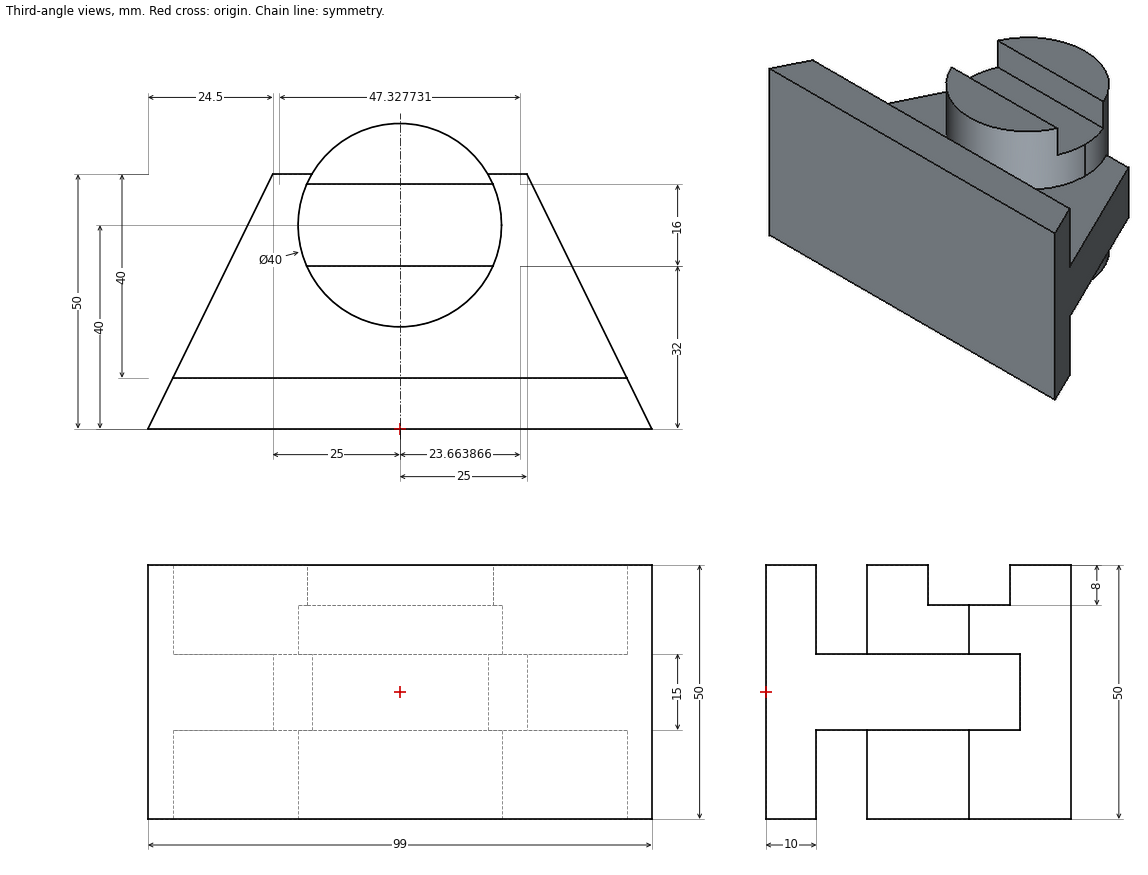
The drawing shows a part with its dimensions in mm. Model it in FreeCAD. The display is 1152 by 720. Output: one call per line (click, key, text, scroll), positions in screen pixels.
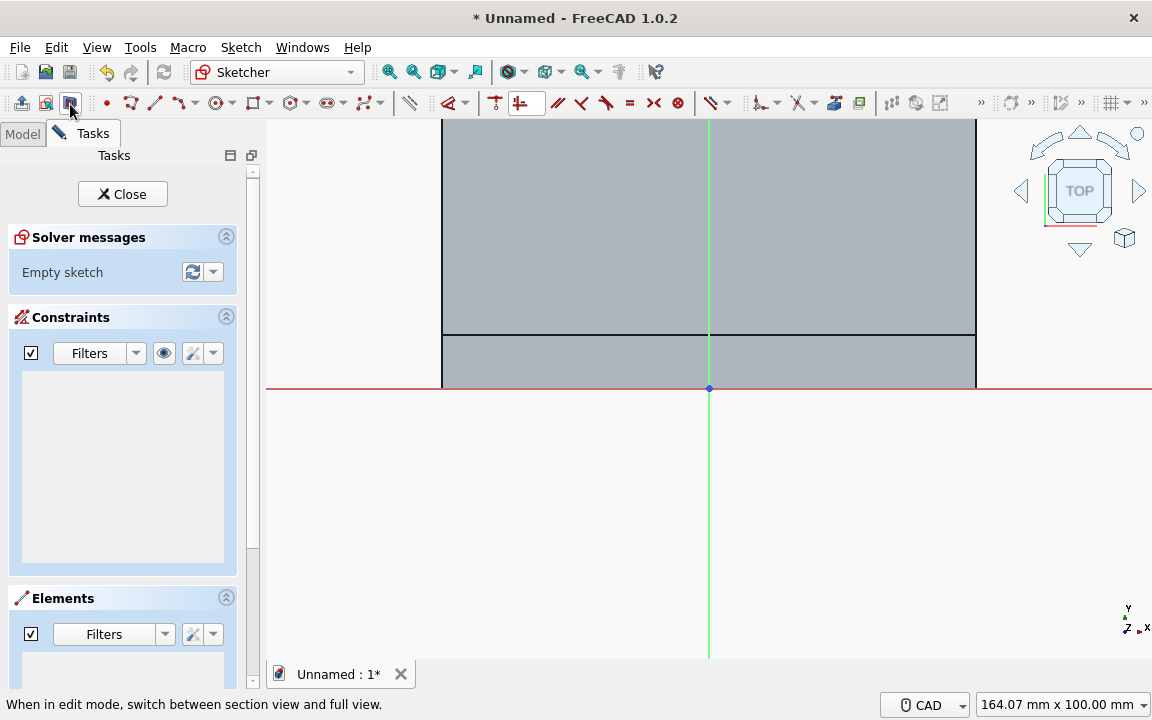
scroll(331, 631, down, 1)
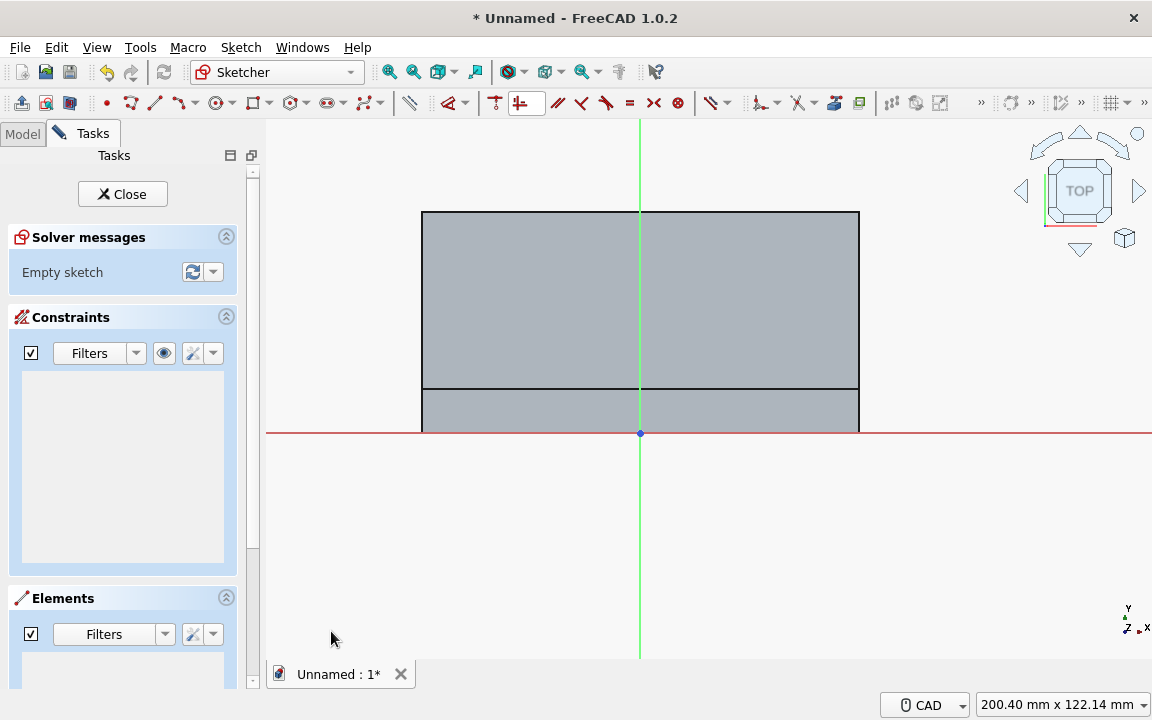
click(132, 104)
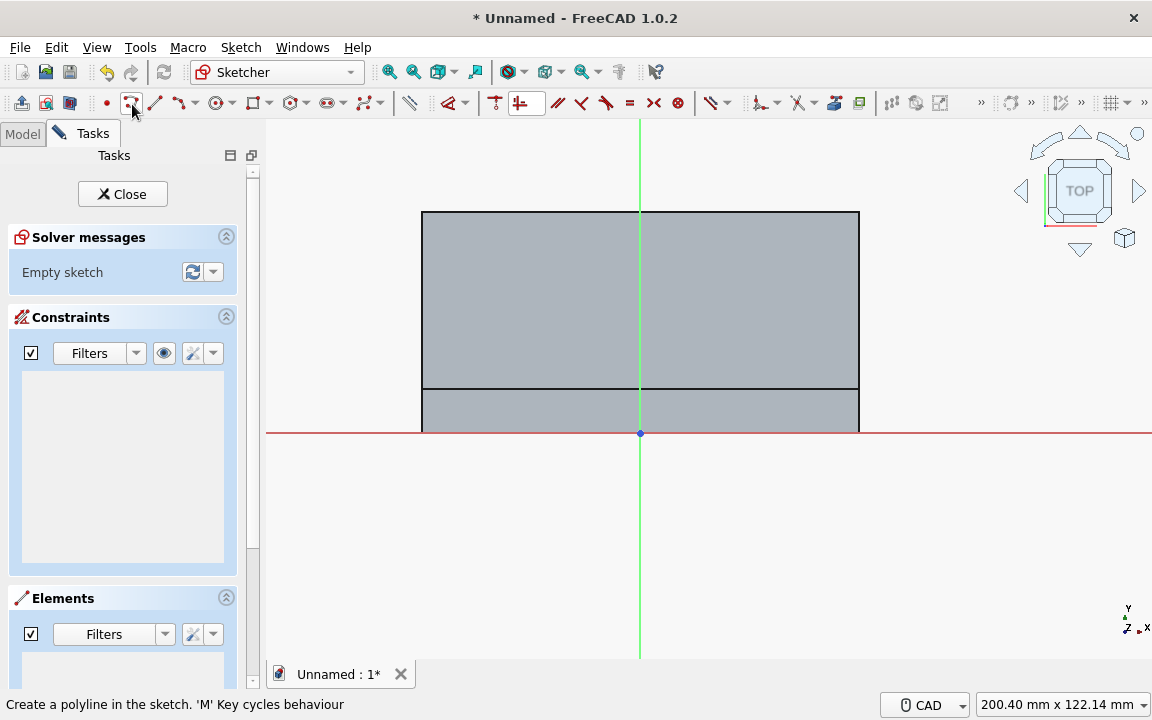
click(422, 433)
click(530, 212)
click(422, 212)
click(422, 433)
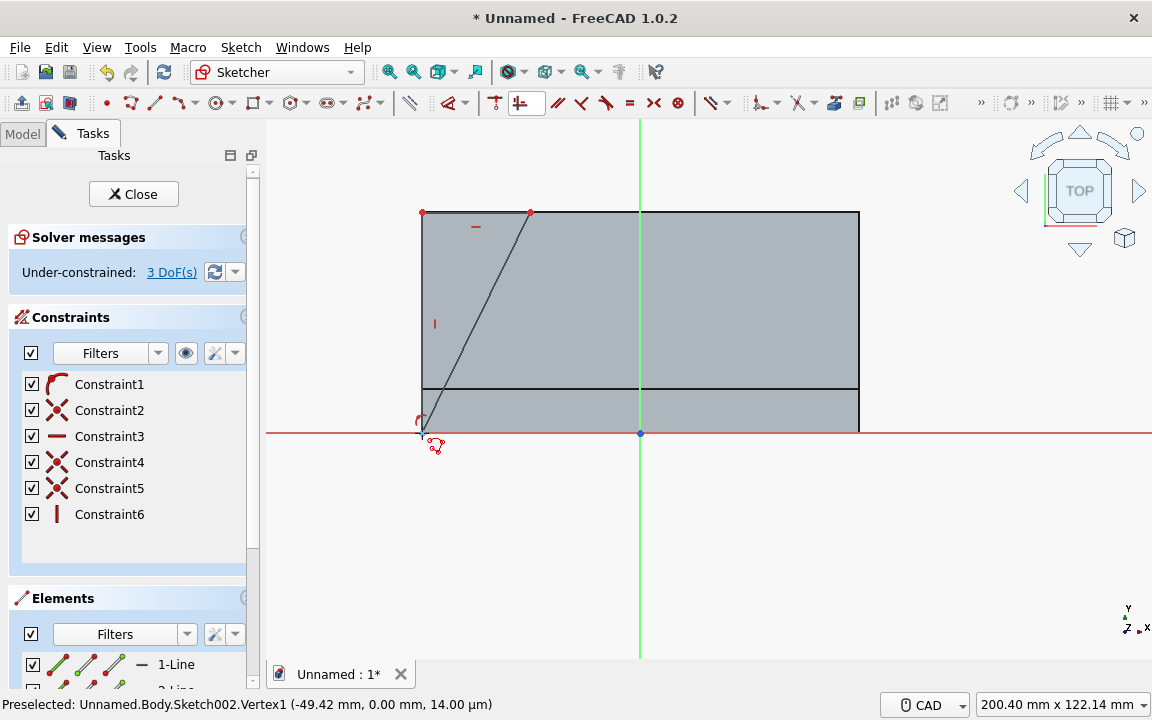
click(859, 433)
click(859, 212)
click(751, 212)
click(859, 433)
key(Escape)
key(Escape)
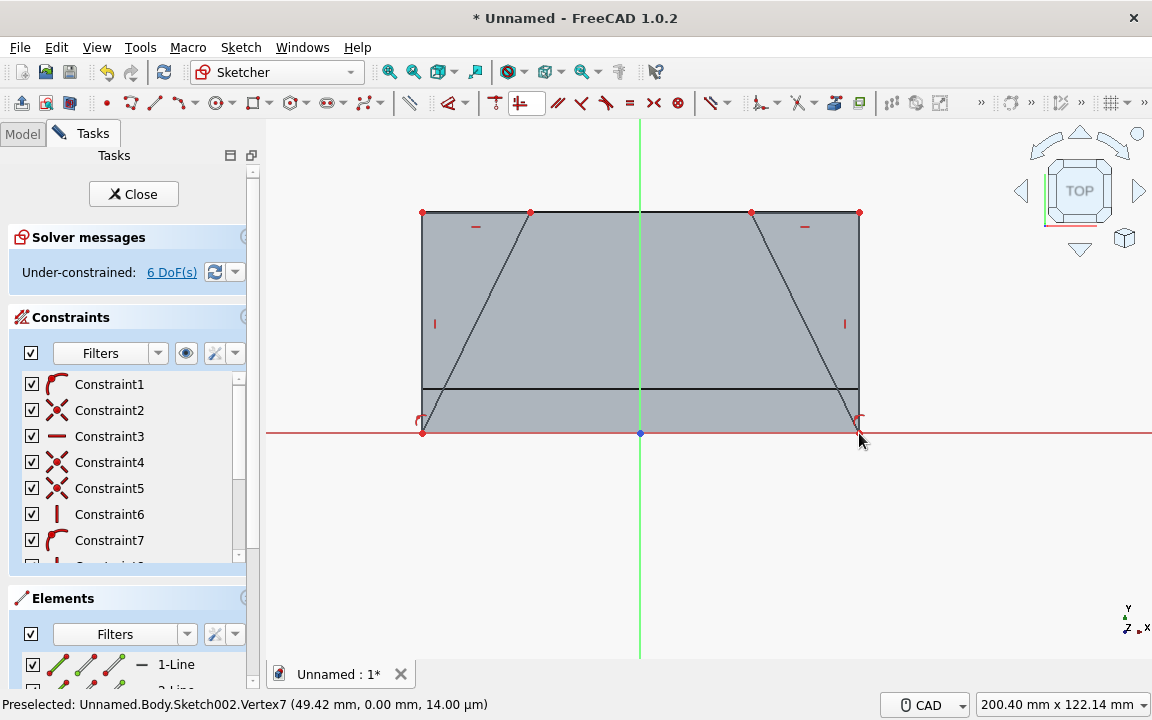
click(422, 213)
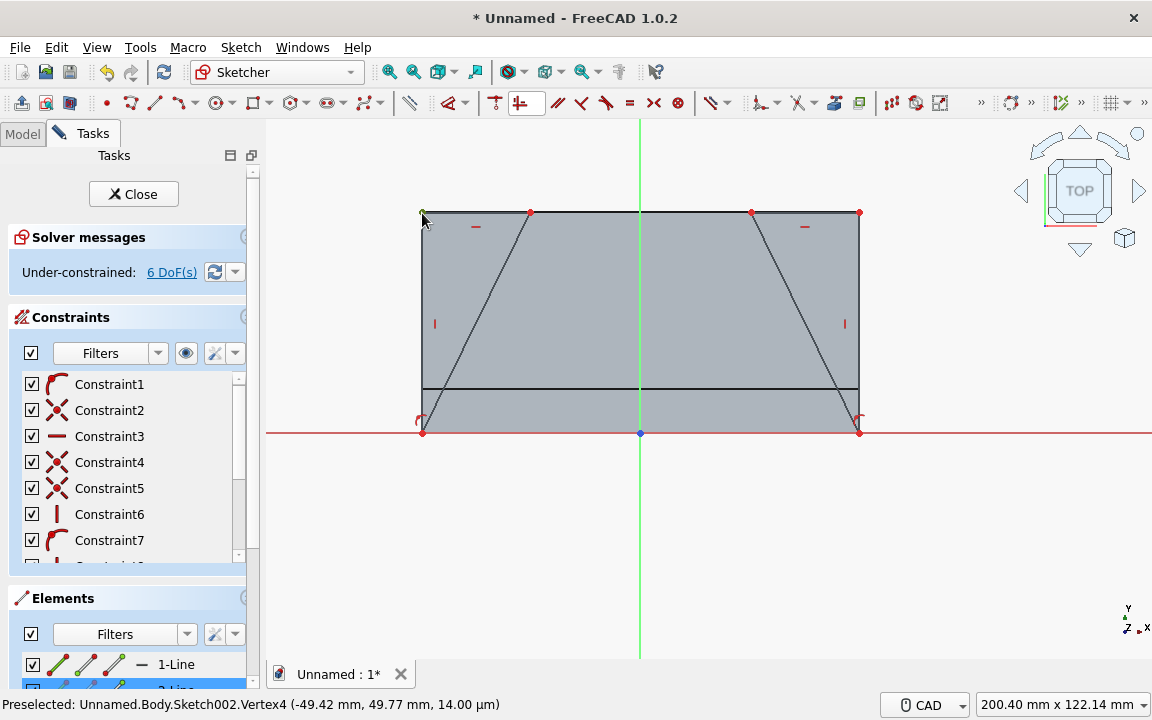
click(859, 213)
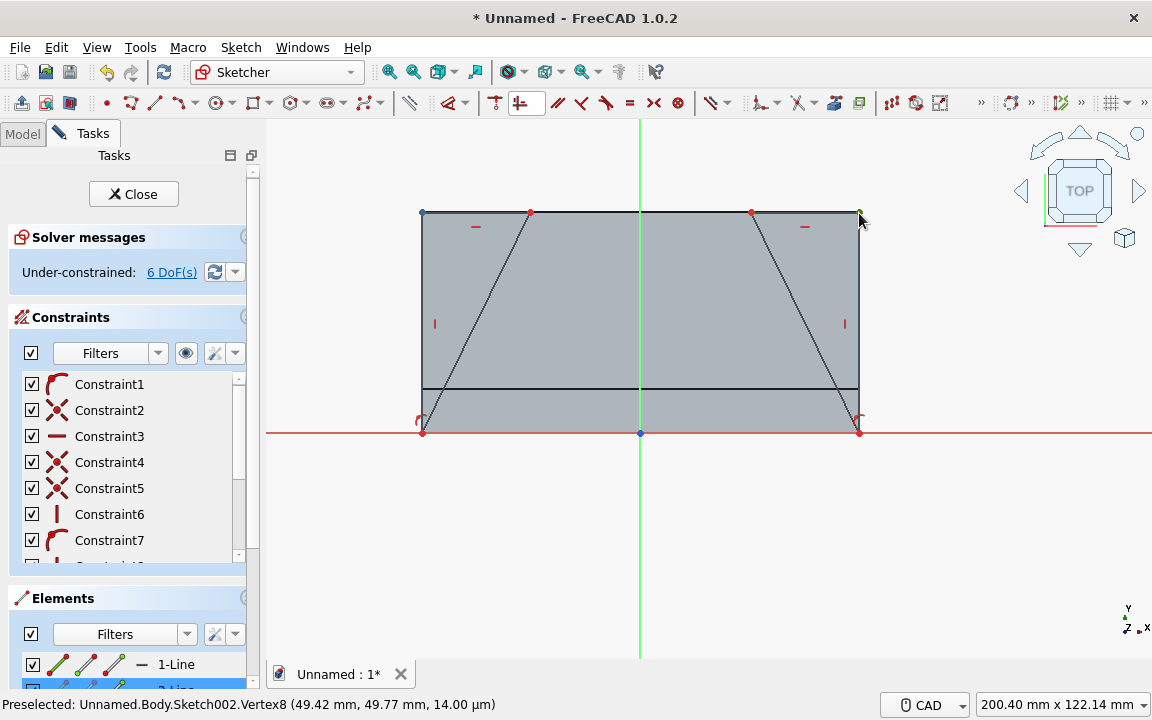
click(640, 596)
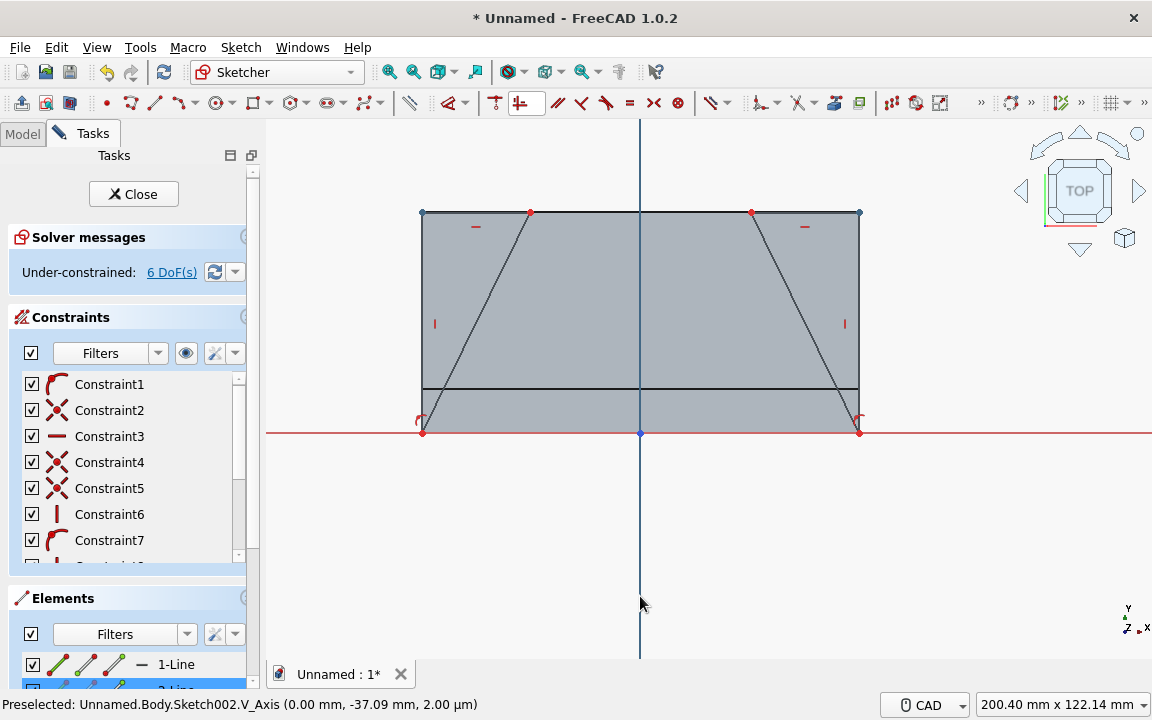
click(654, 104)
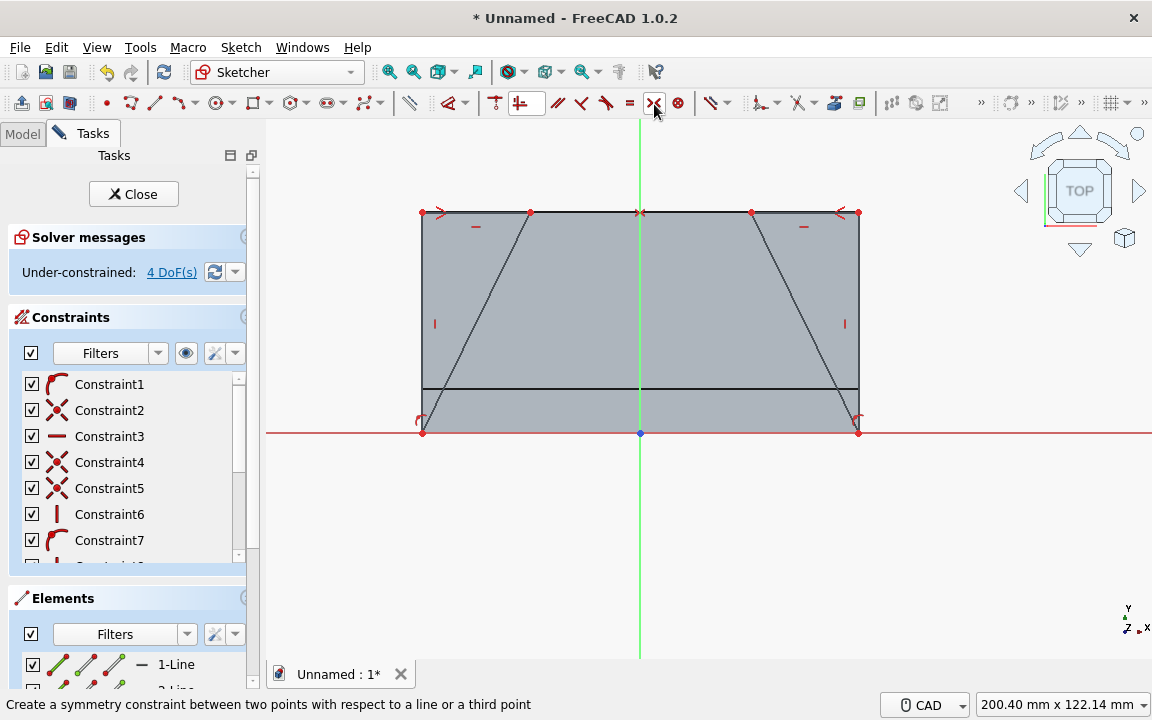
key(d)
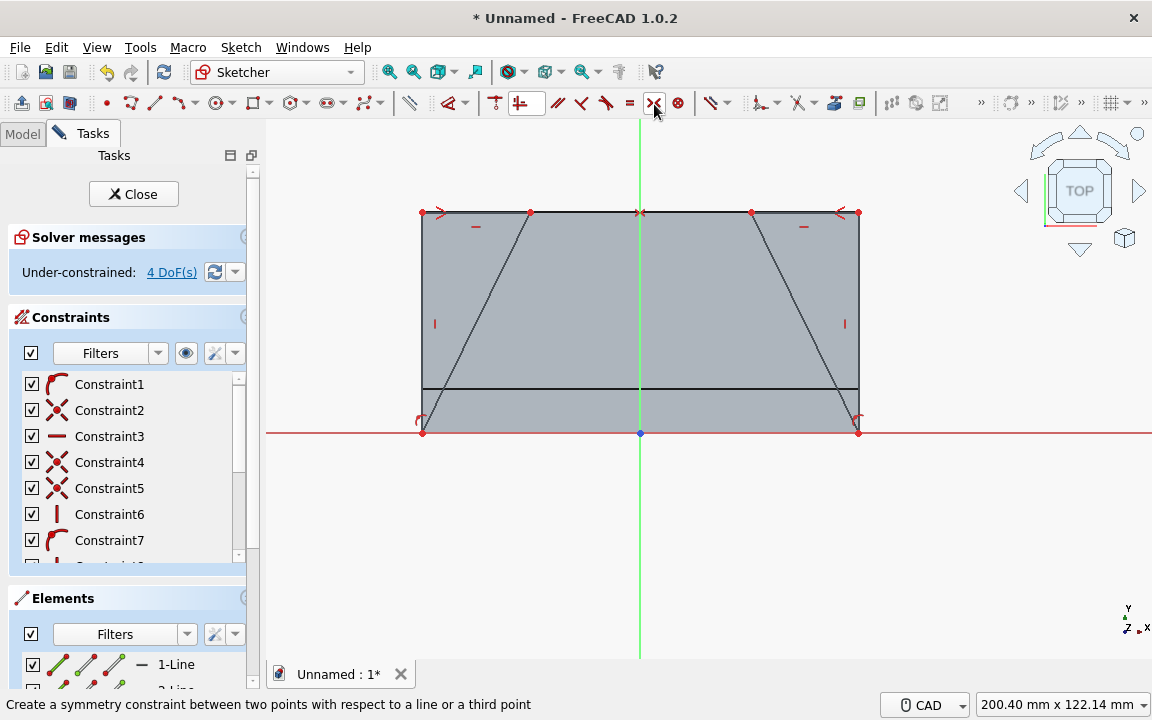
click(422, 279)
click(388, 323)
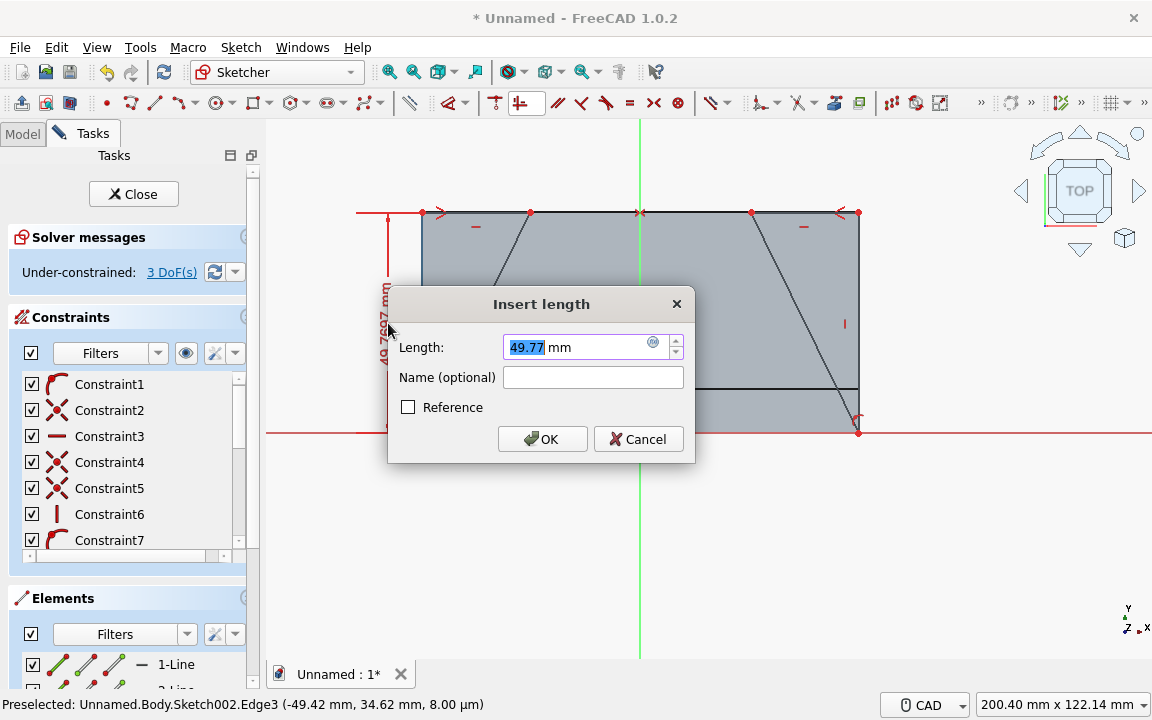
text(50)
key(Return)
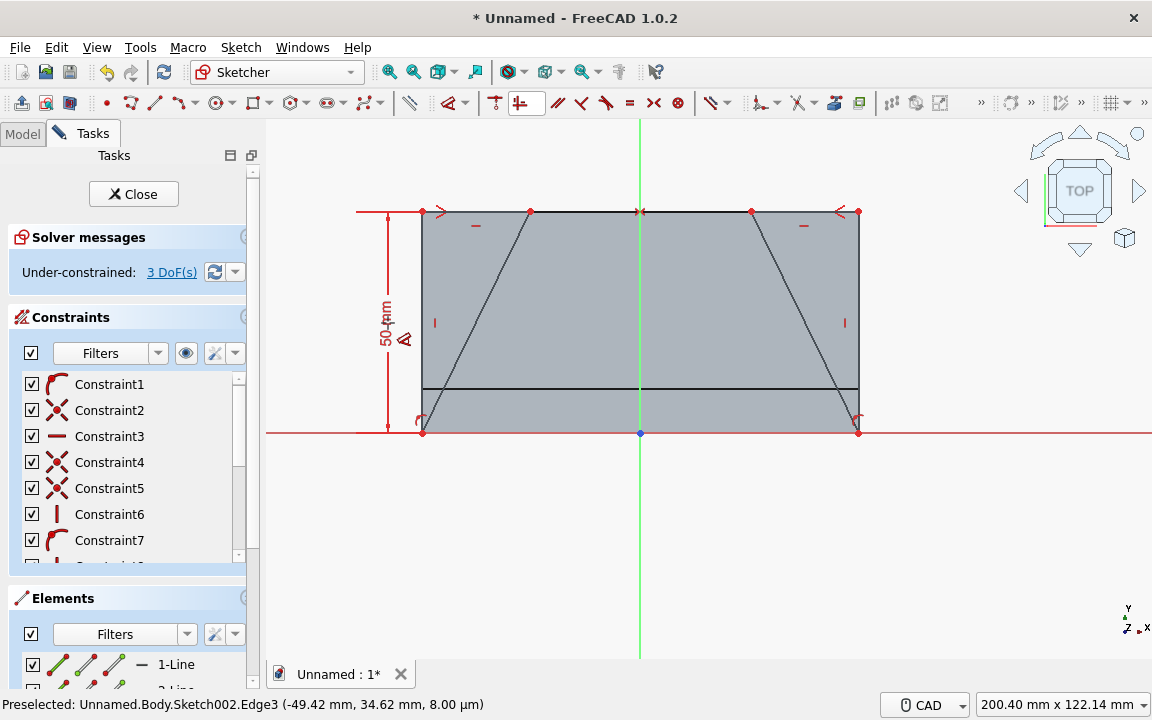
click(530, 212)
click(585, 467)